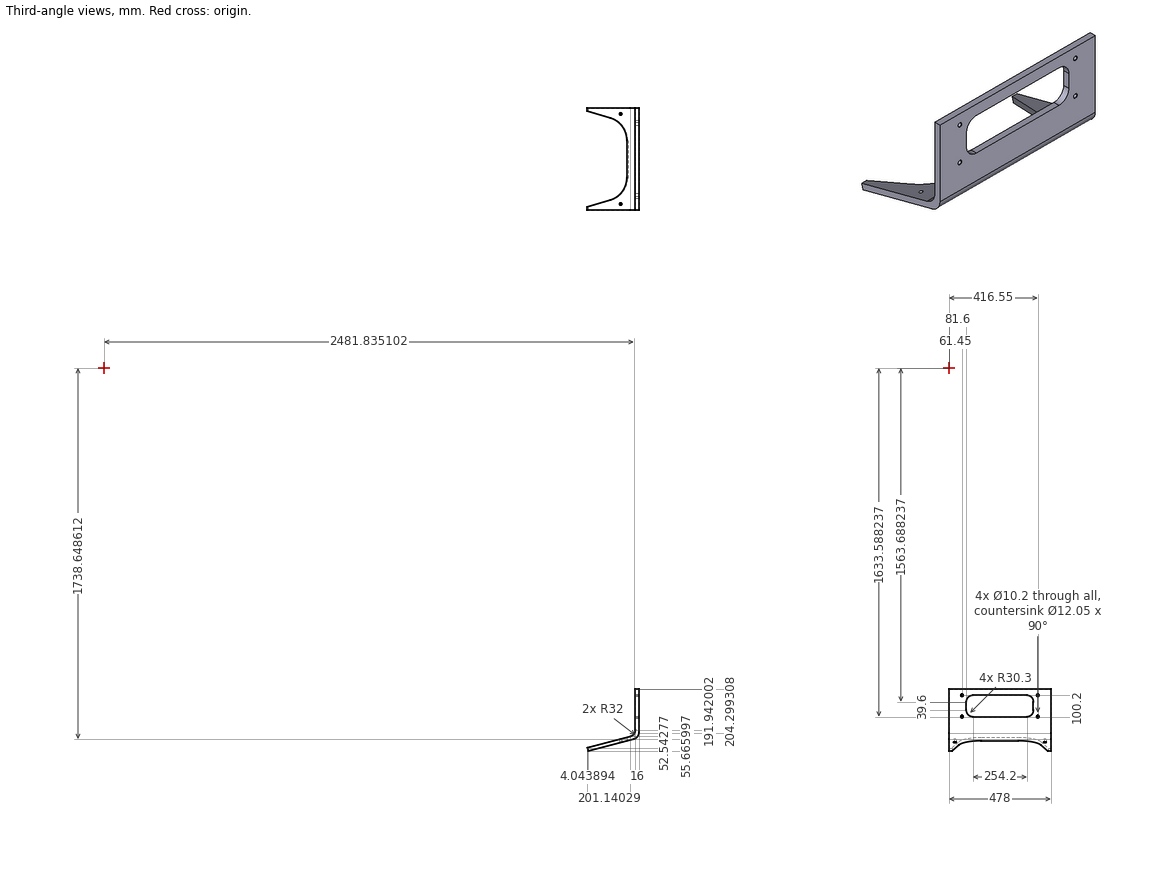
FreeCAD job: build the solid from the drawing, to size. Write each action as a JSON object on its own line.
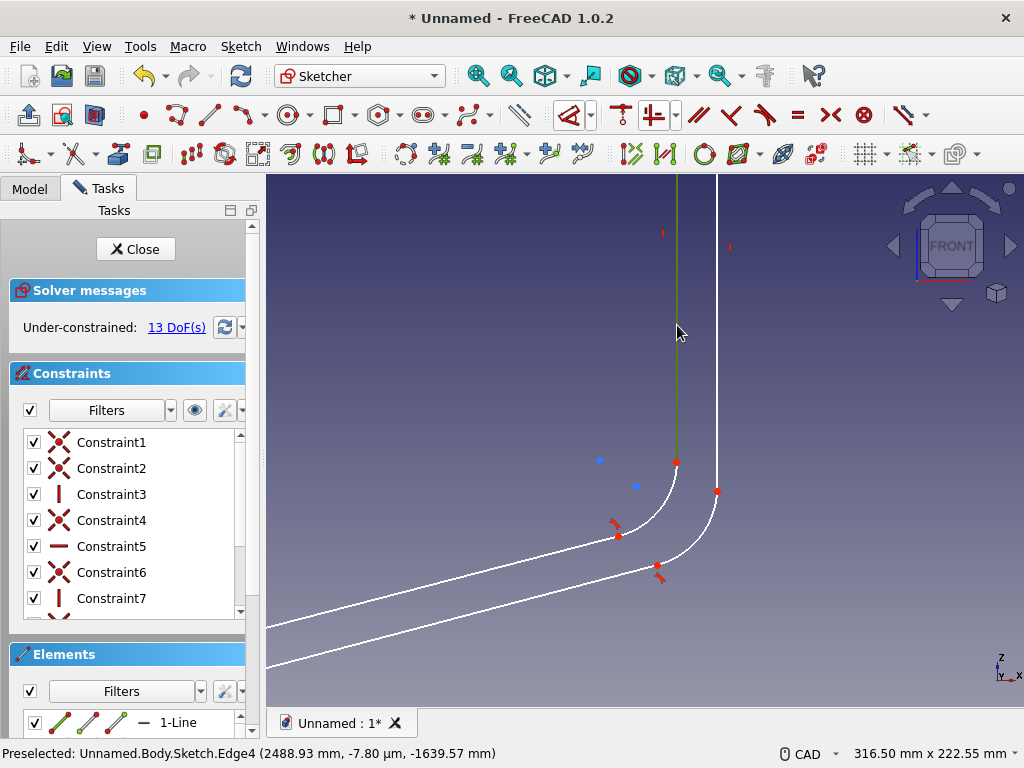
{"action": "left_click", "coordinate": [646, 523]}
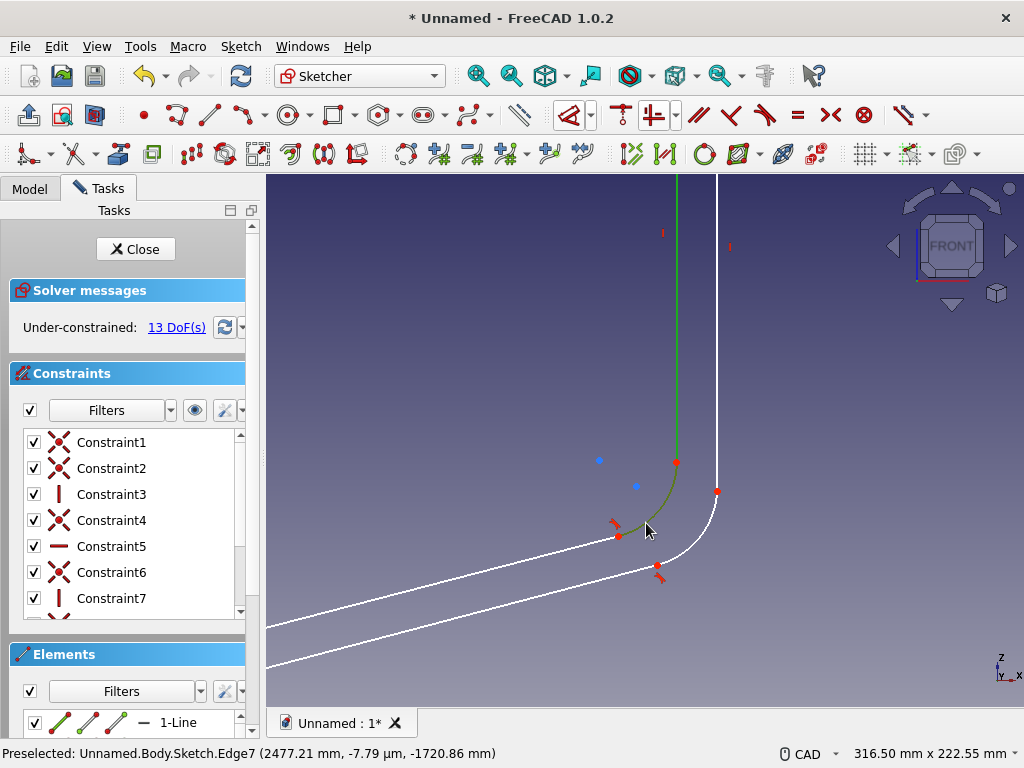
{"action": "left_click", "coordinate": [765, 116]}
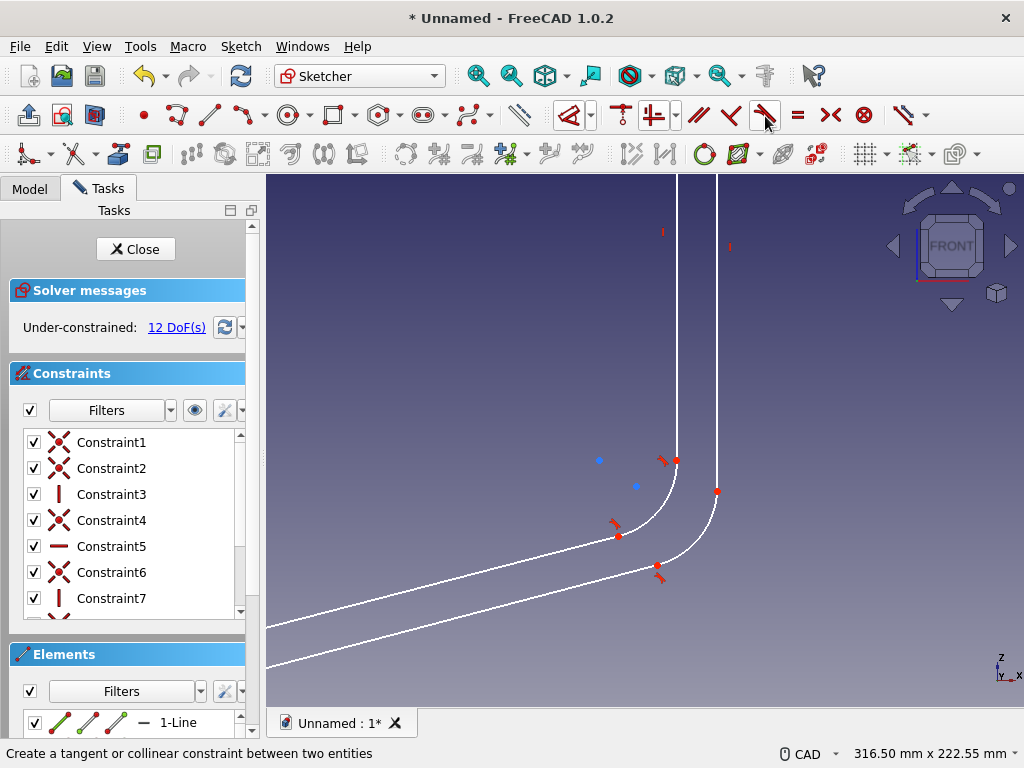
{"action": "left_click", "coordinate": [717, 345]}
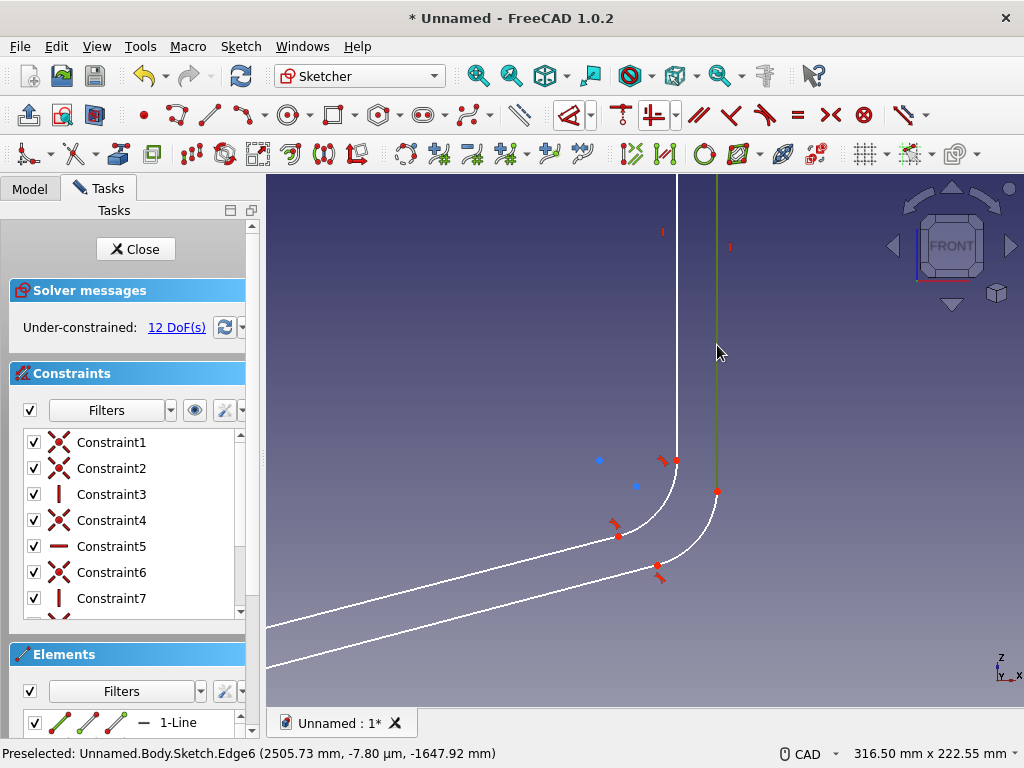
{"action": "left_click", "coordinate": [684, 552]}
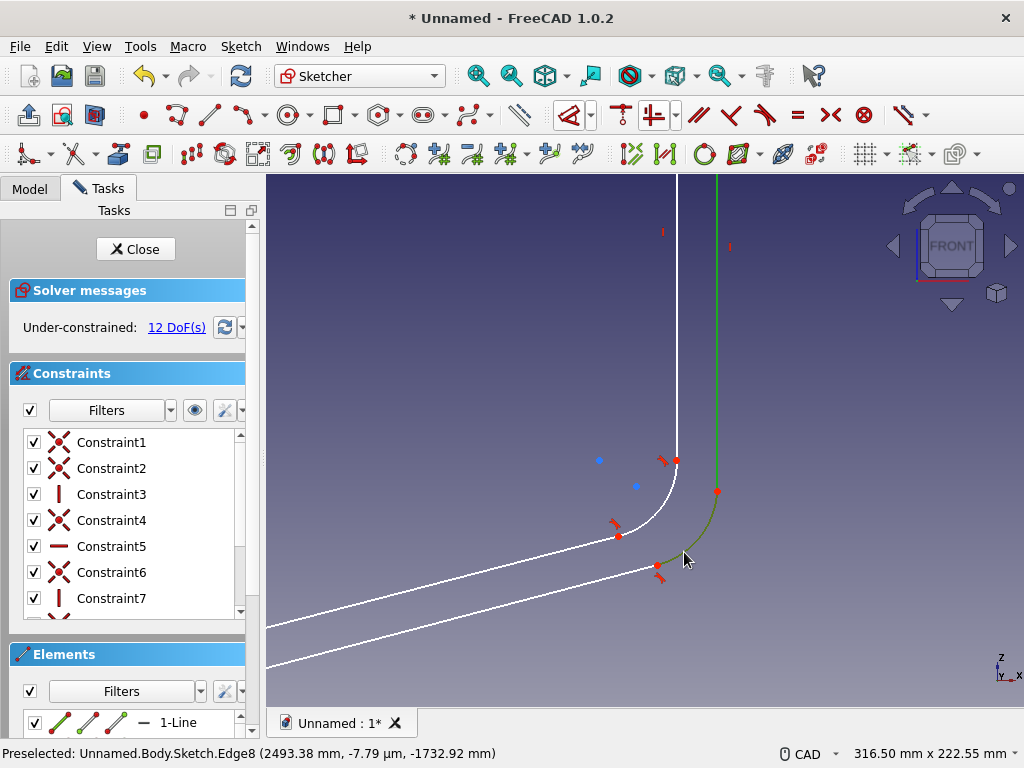
{"action": "left_click", "coordinate": [765, 116]}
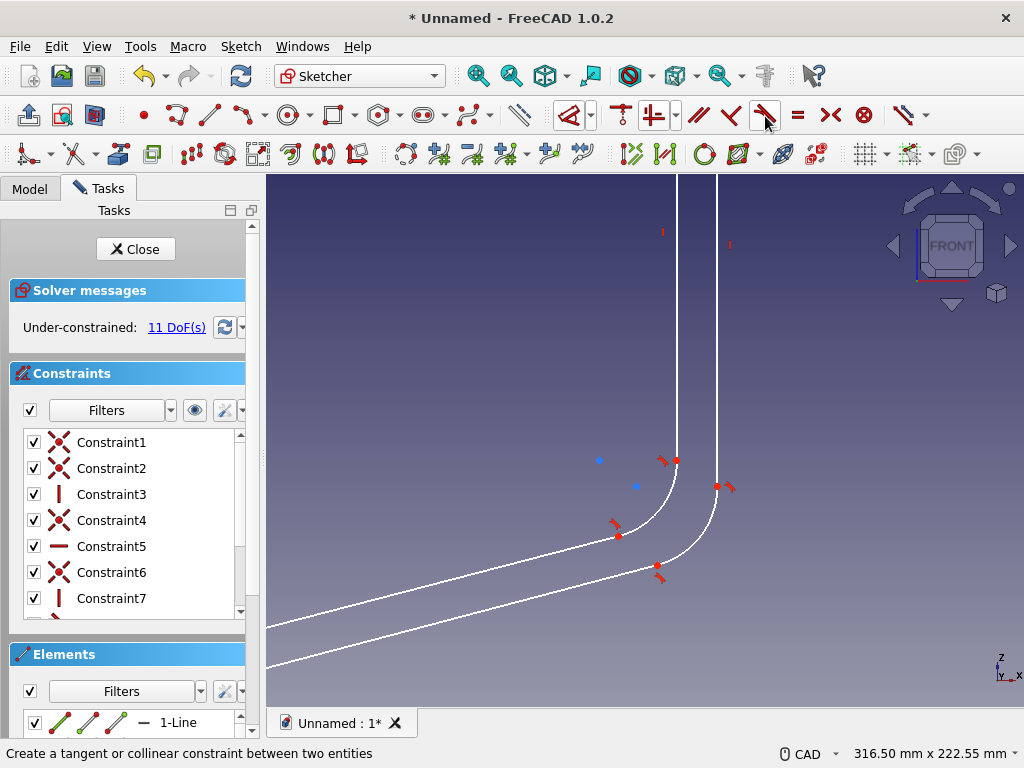
{"action": "left_click", "coordinate": [646, 523]}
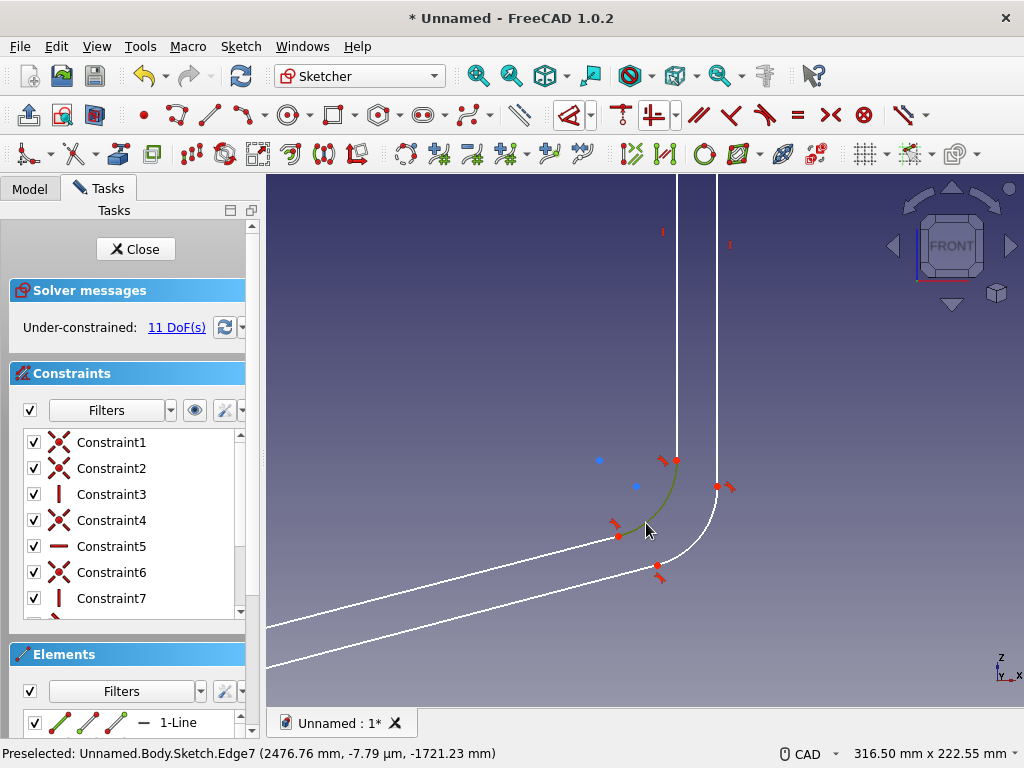
{"action": "left_click", "coordinate": [686, 551]}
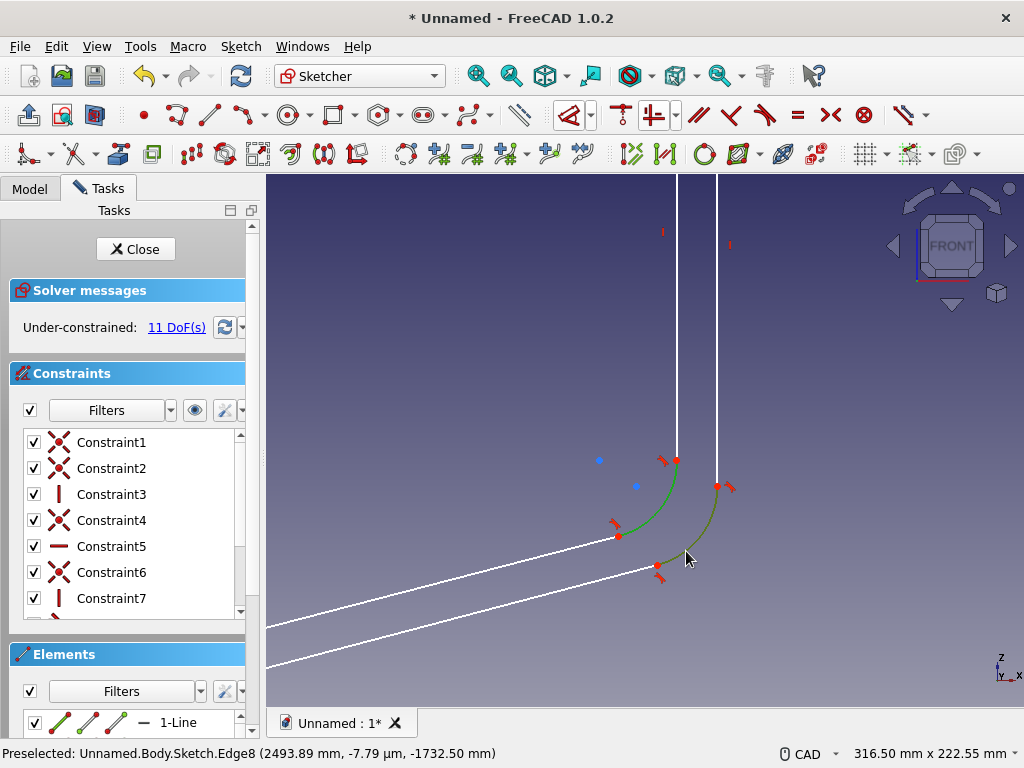
{"action": "left_click", "coordinate": [798, 116]}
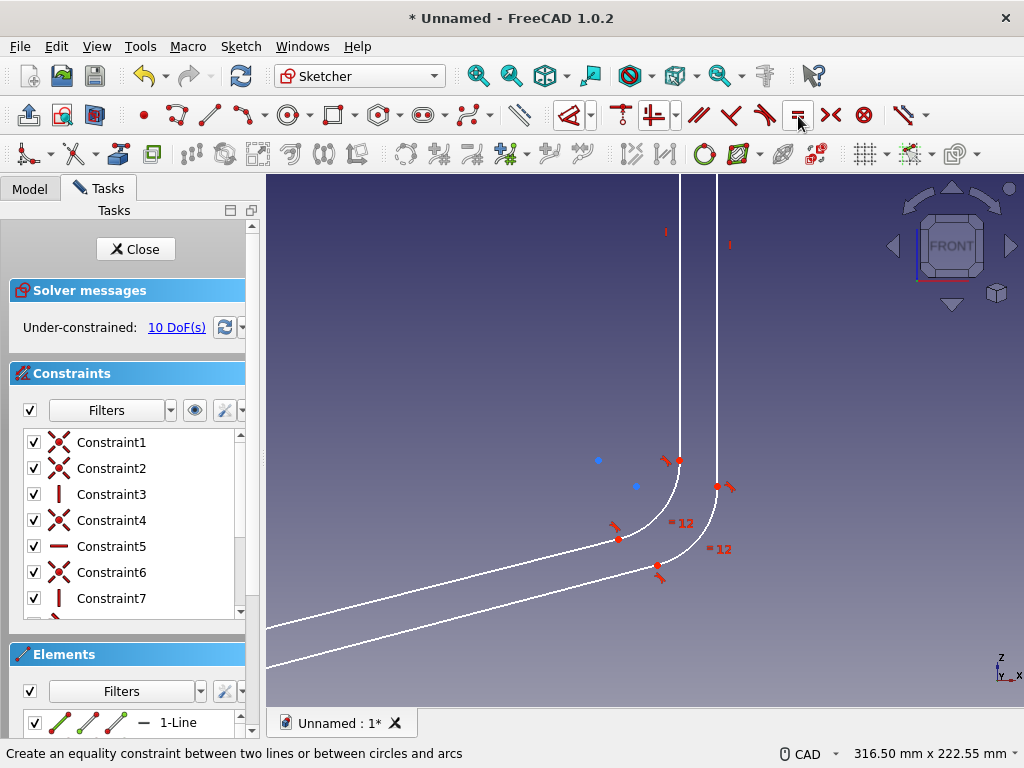
{"action": "left_click", "coordinate": [568, 116]}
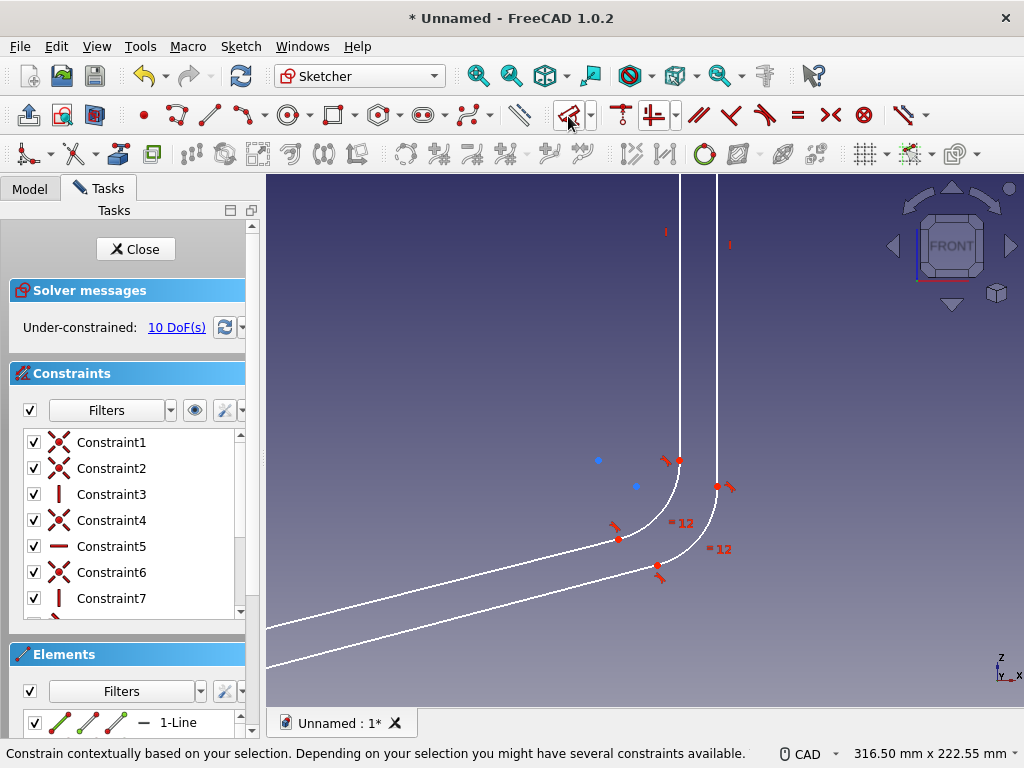
{"action": "left_click", "coordinate": [648, 525]}
{"action": "left_click", "coordinate": [509, 529]}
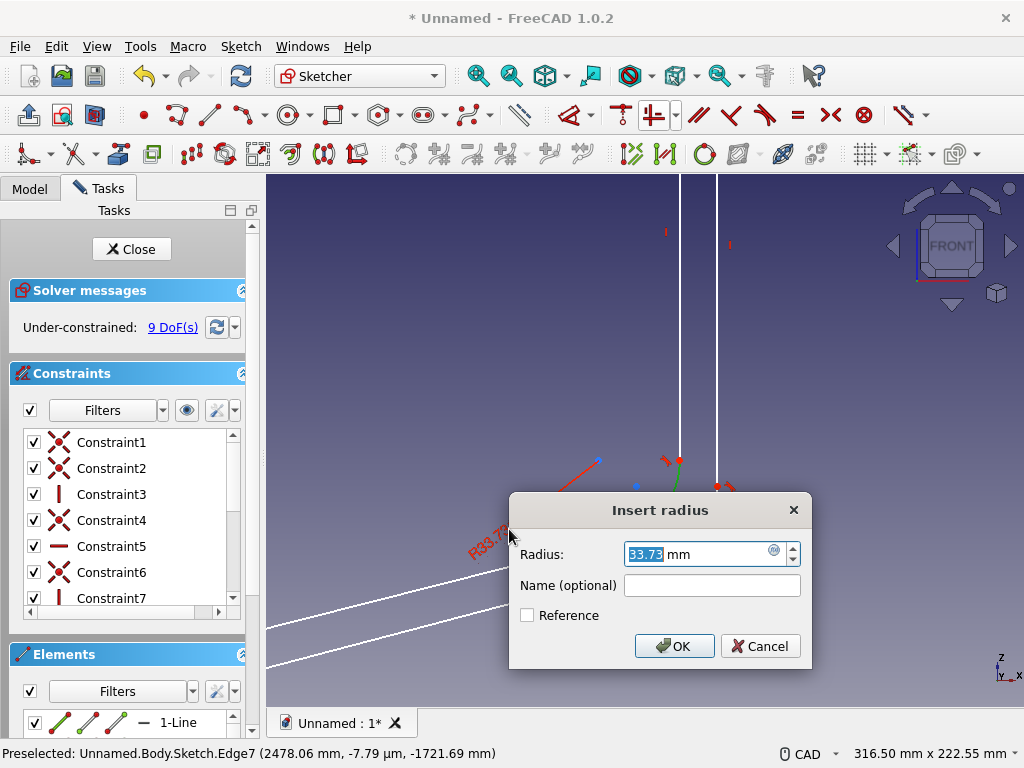
{"action": "type", "text": "32"}
{"action": "key", "text": "Return"}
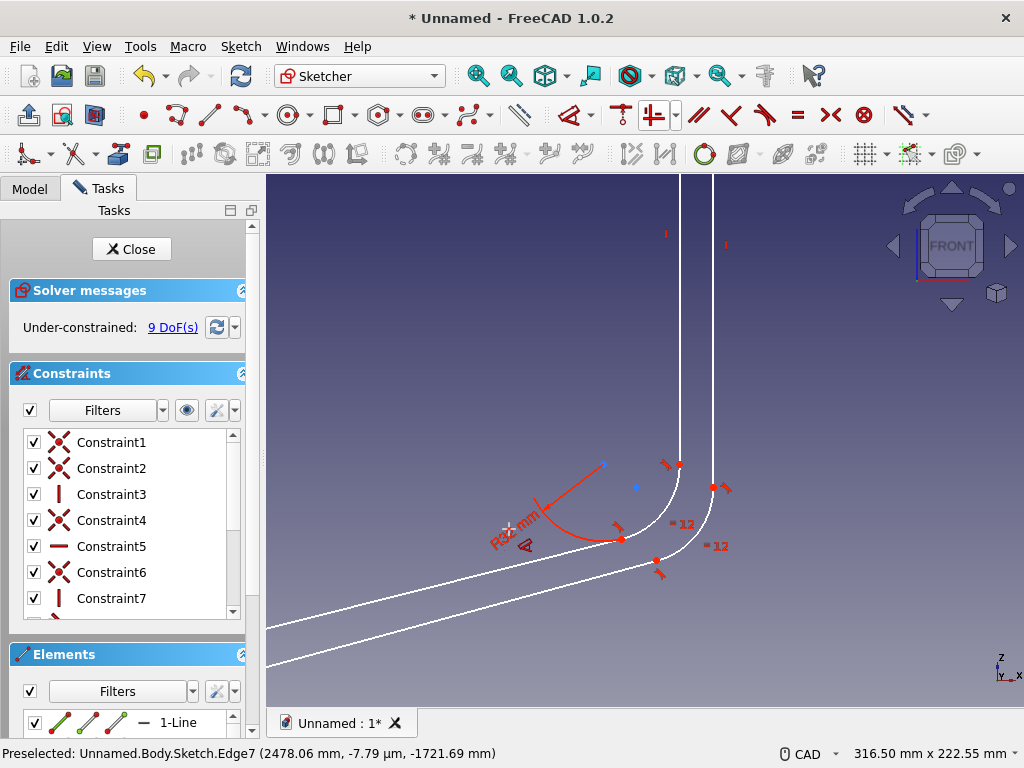
{"action": "scroll", "coordinate": [697, 516], "scroll_direction": "down", "scroll_amount": 4}